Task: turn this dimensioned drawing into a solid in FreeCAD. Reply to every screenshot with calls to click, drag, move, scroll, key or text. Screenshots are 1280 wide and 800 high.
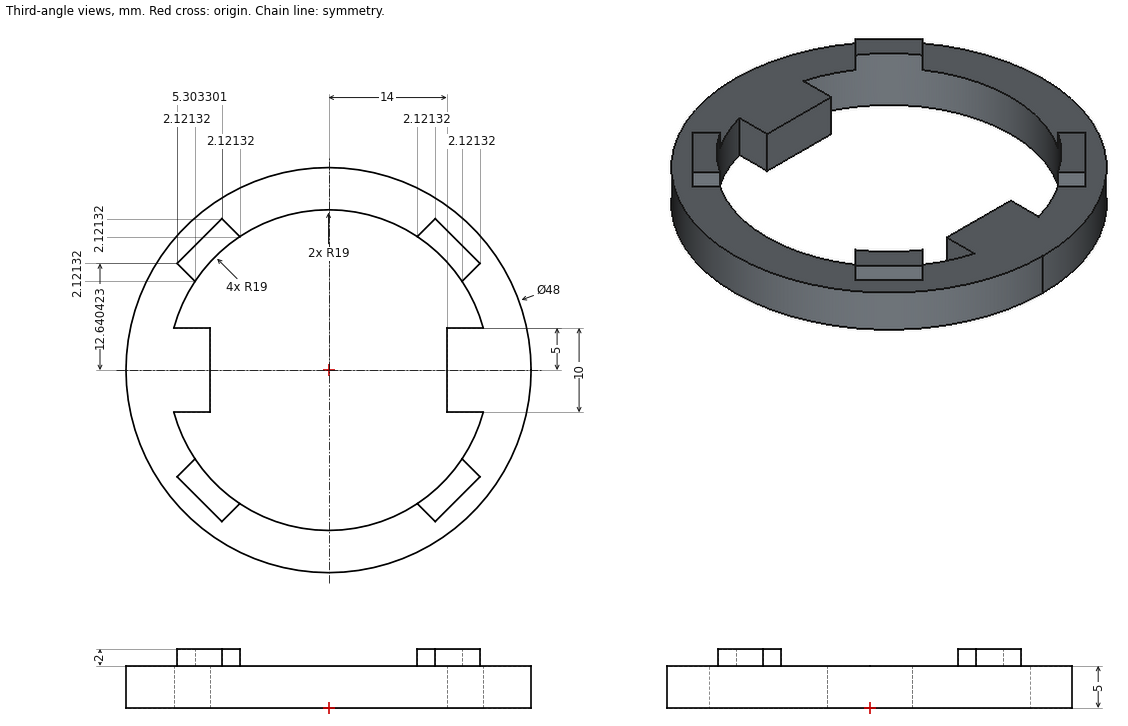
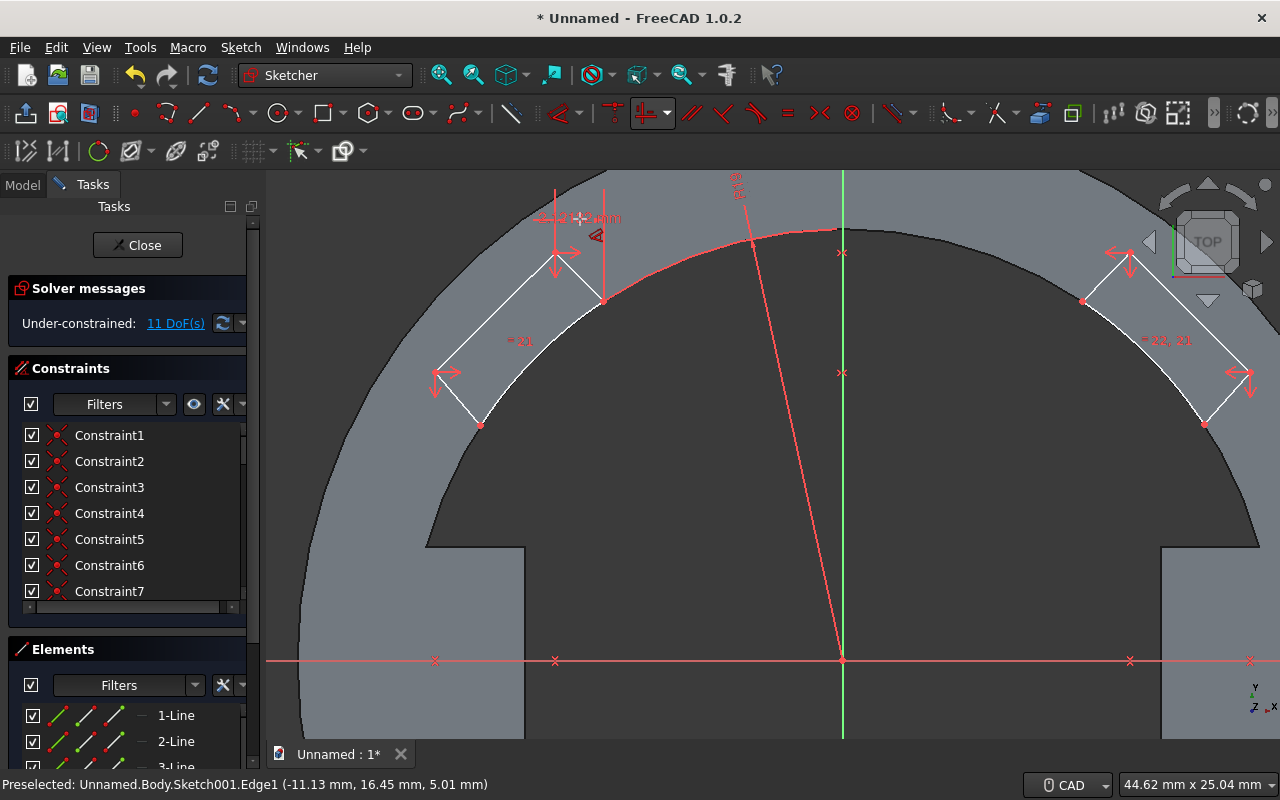
click(589, 287)
click(521, 266)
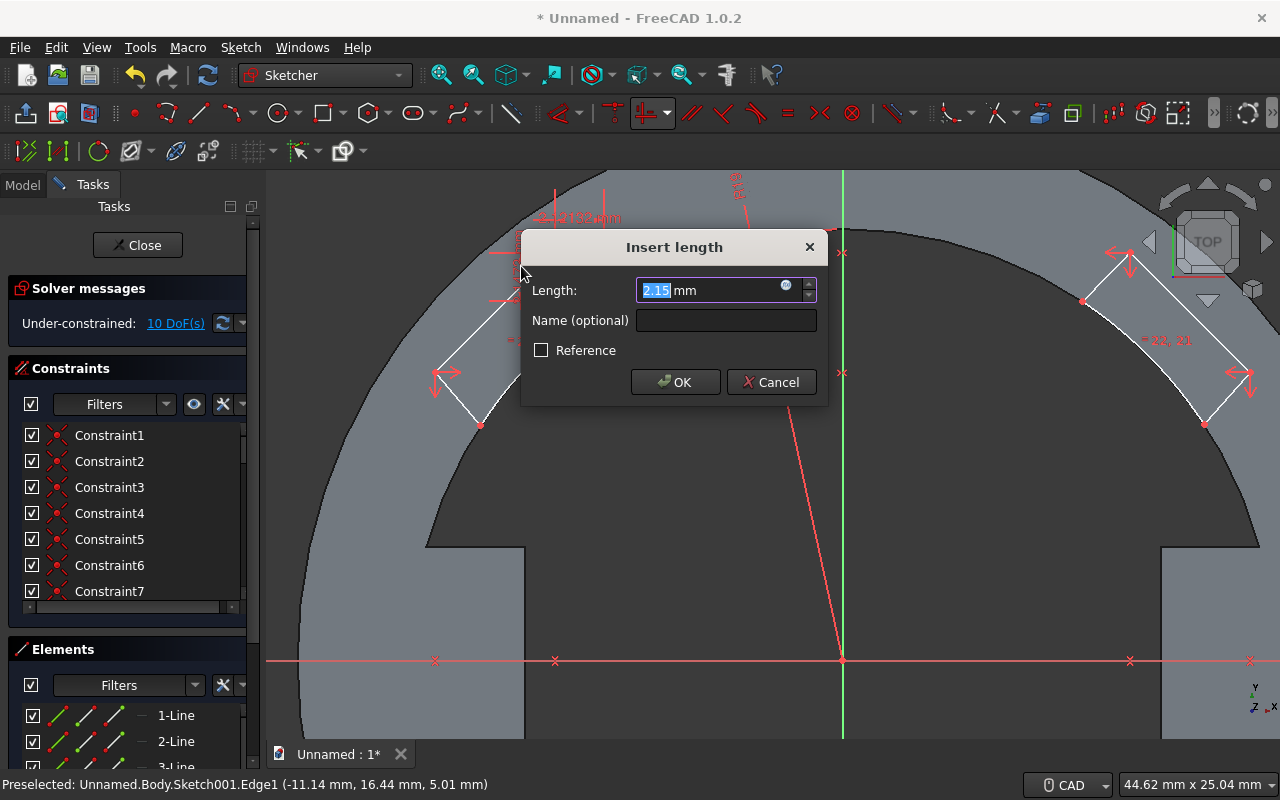
text(2.12132)
key(Return)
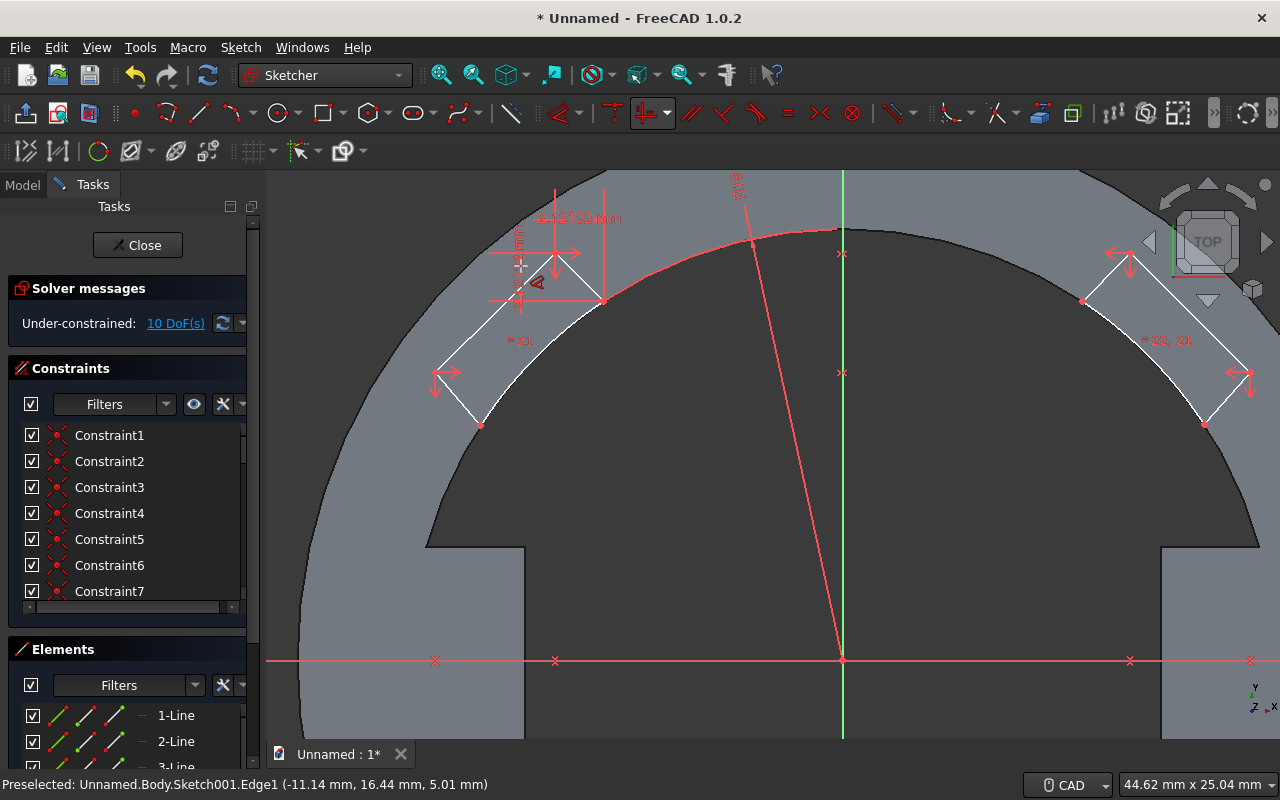
click(449, 388)
click(448, 338)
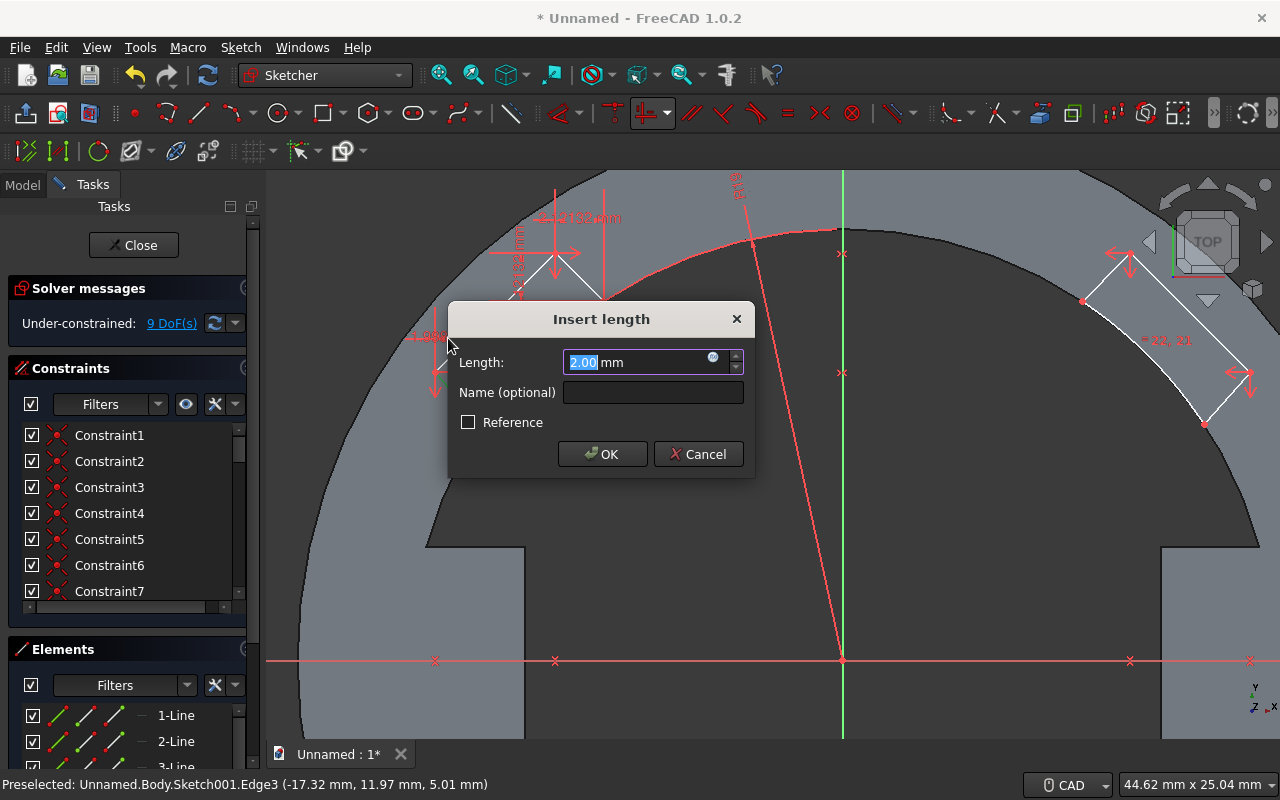
text(2.12132)
key(Return)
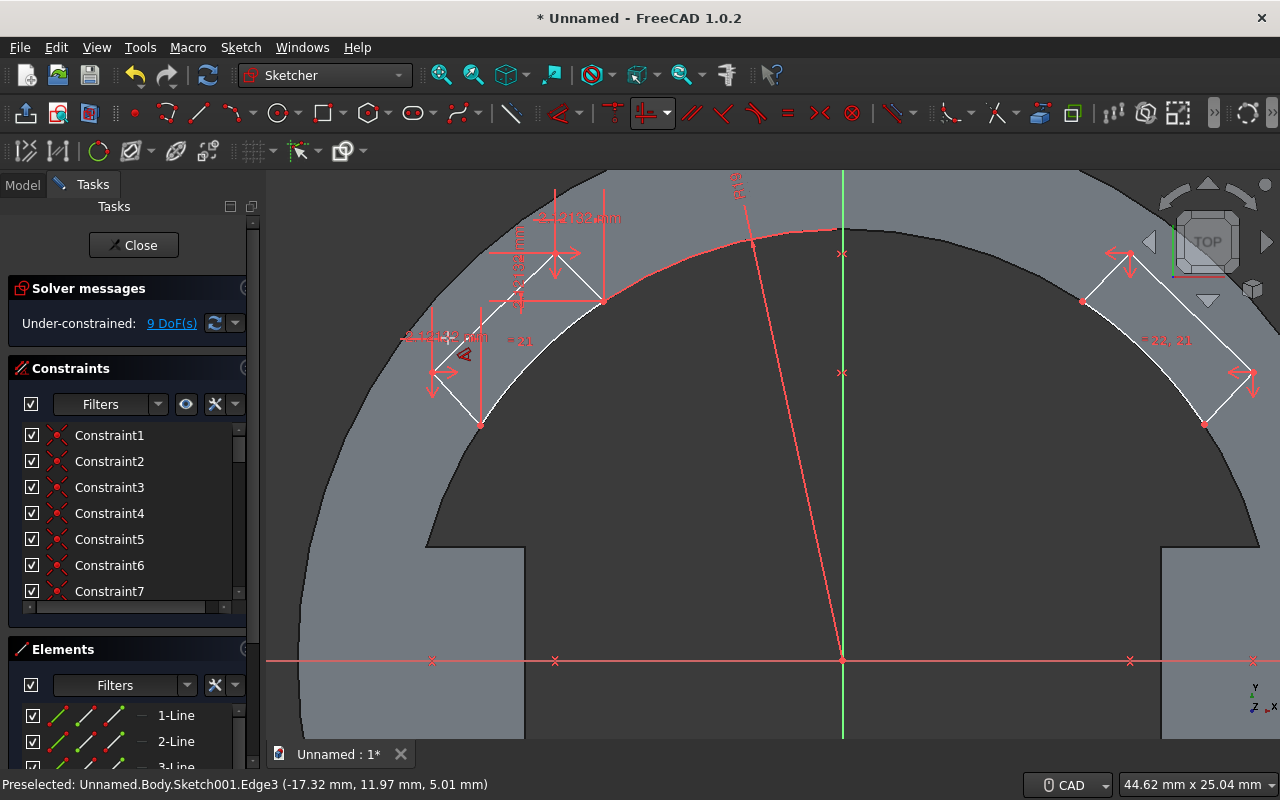
click(447, 388)
click(398, 399)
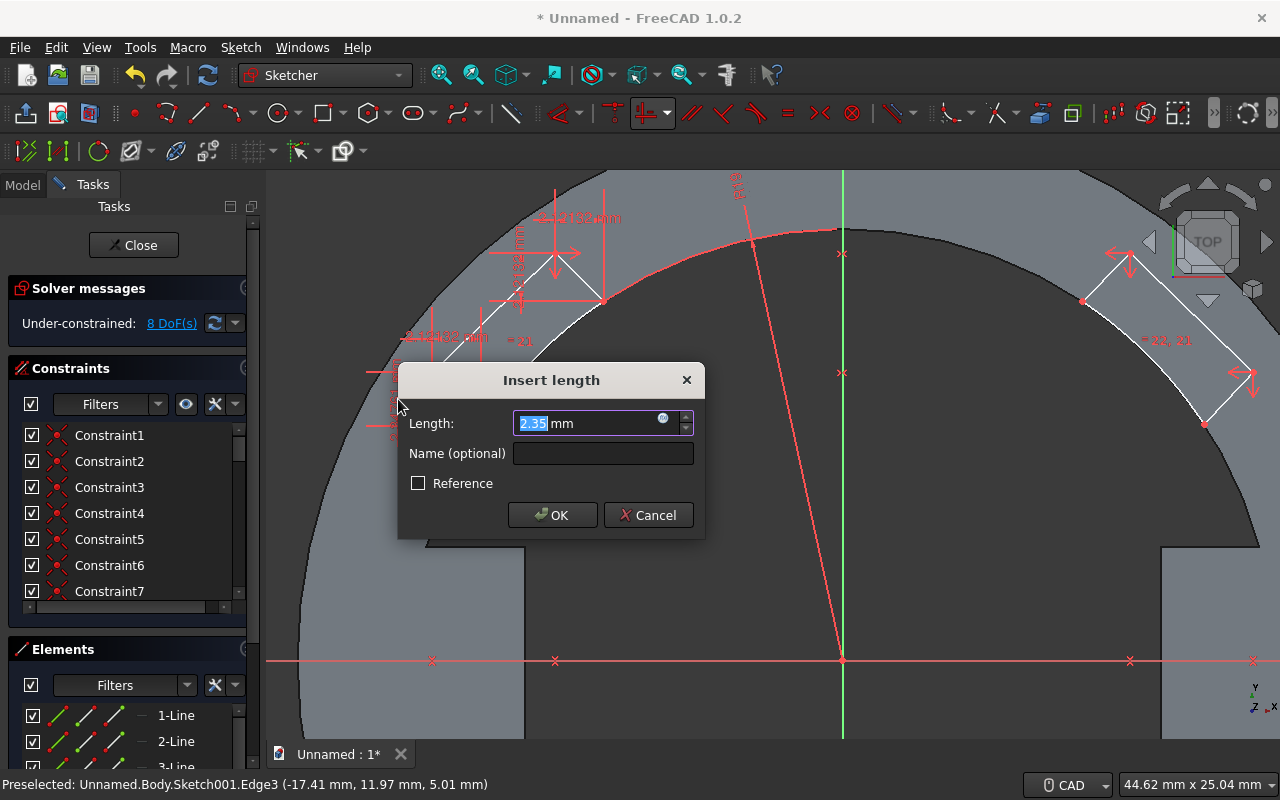
text(2.12132)
key(Return)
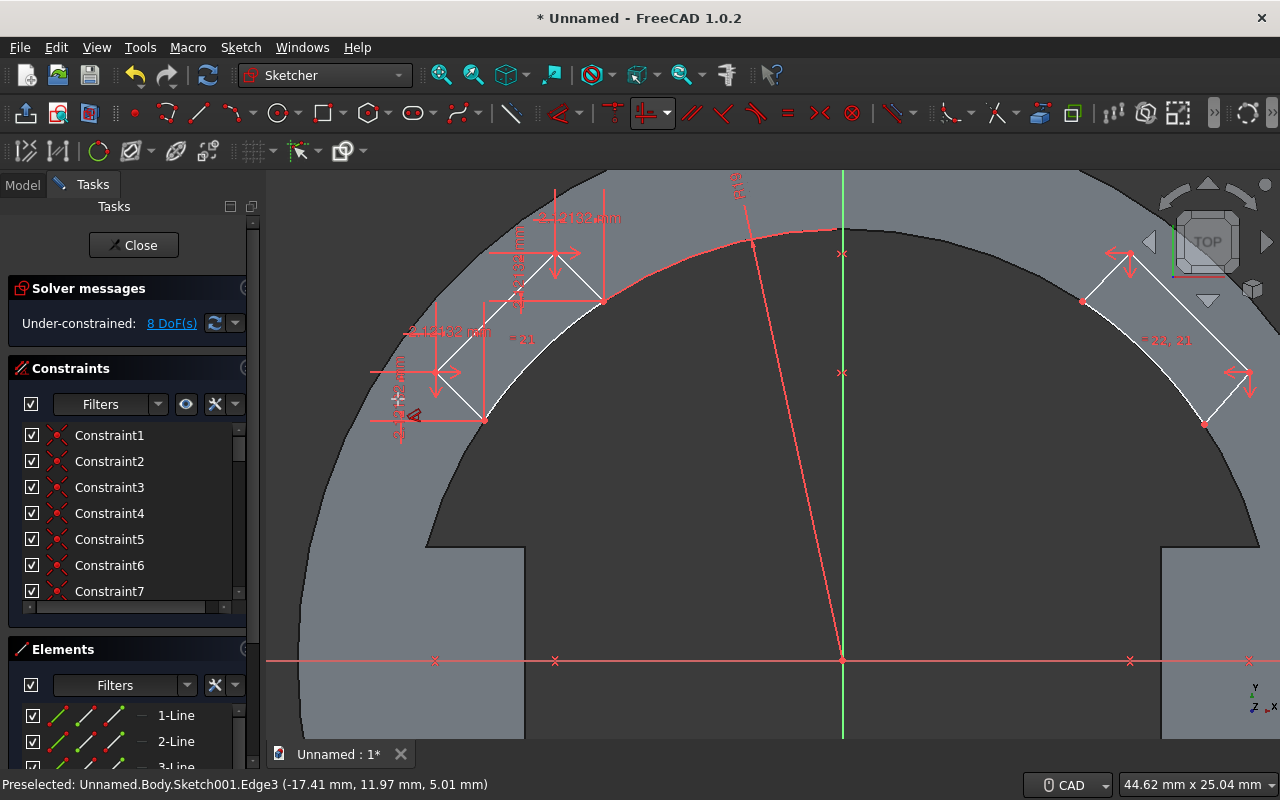
scroll(592, 286, down, 4)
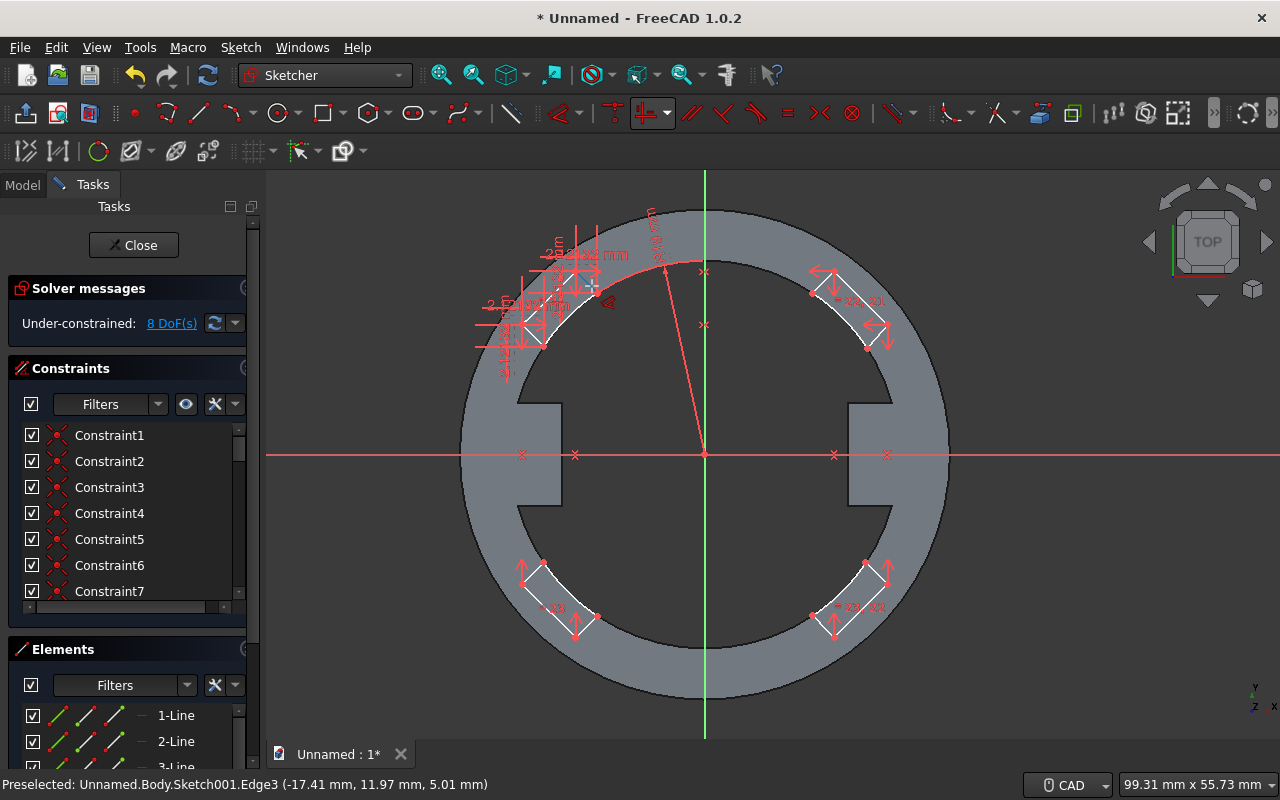
scroll(873, 341, up, 4)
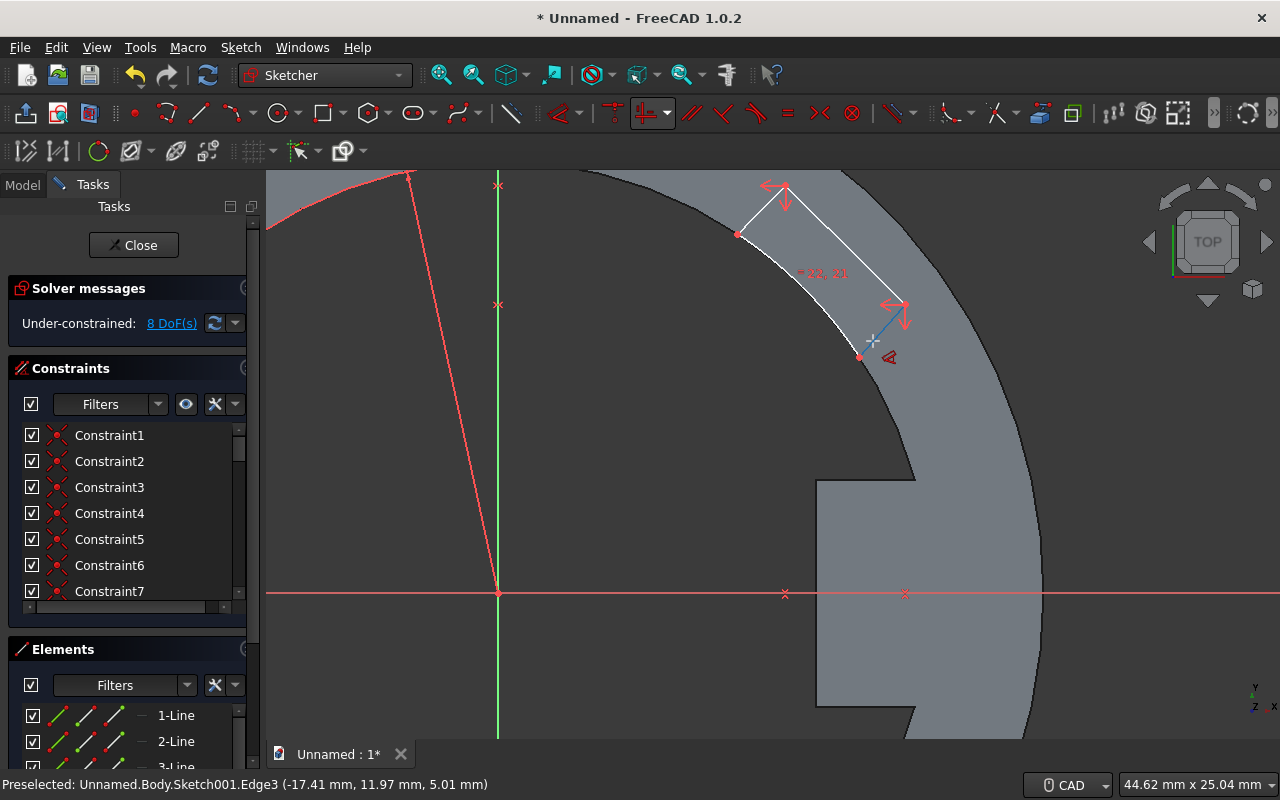
click(873, 341)
click(893, 271)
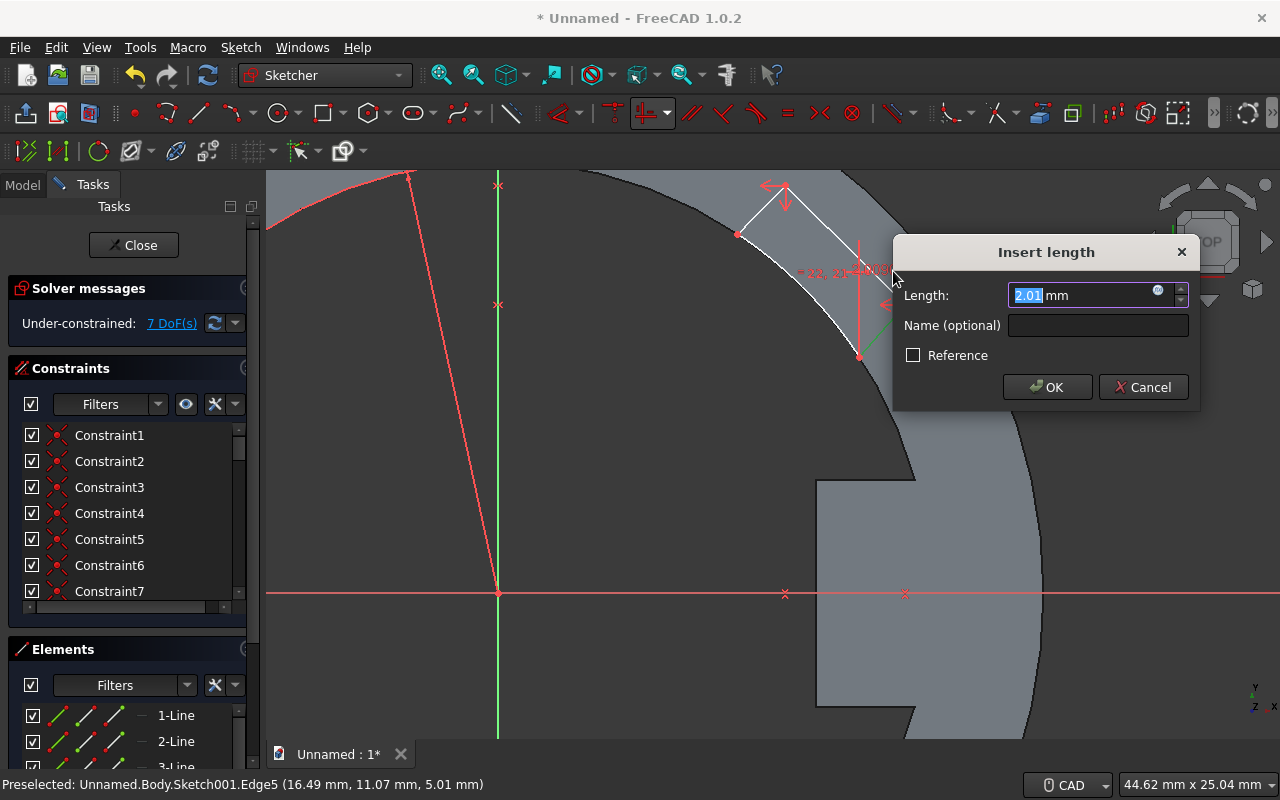
text(2.12132)
key(Return)